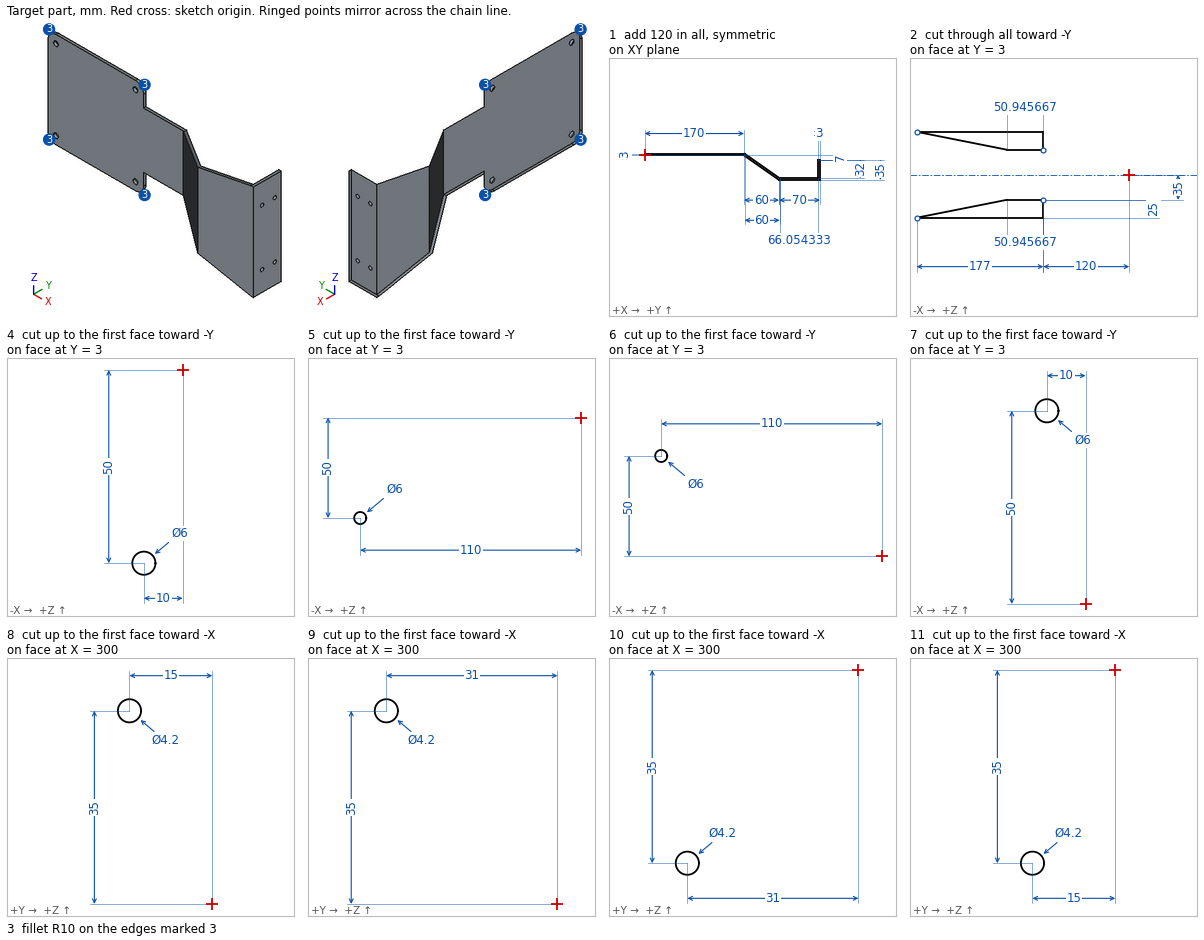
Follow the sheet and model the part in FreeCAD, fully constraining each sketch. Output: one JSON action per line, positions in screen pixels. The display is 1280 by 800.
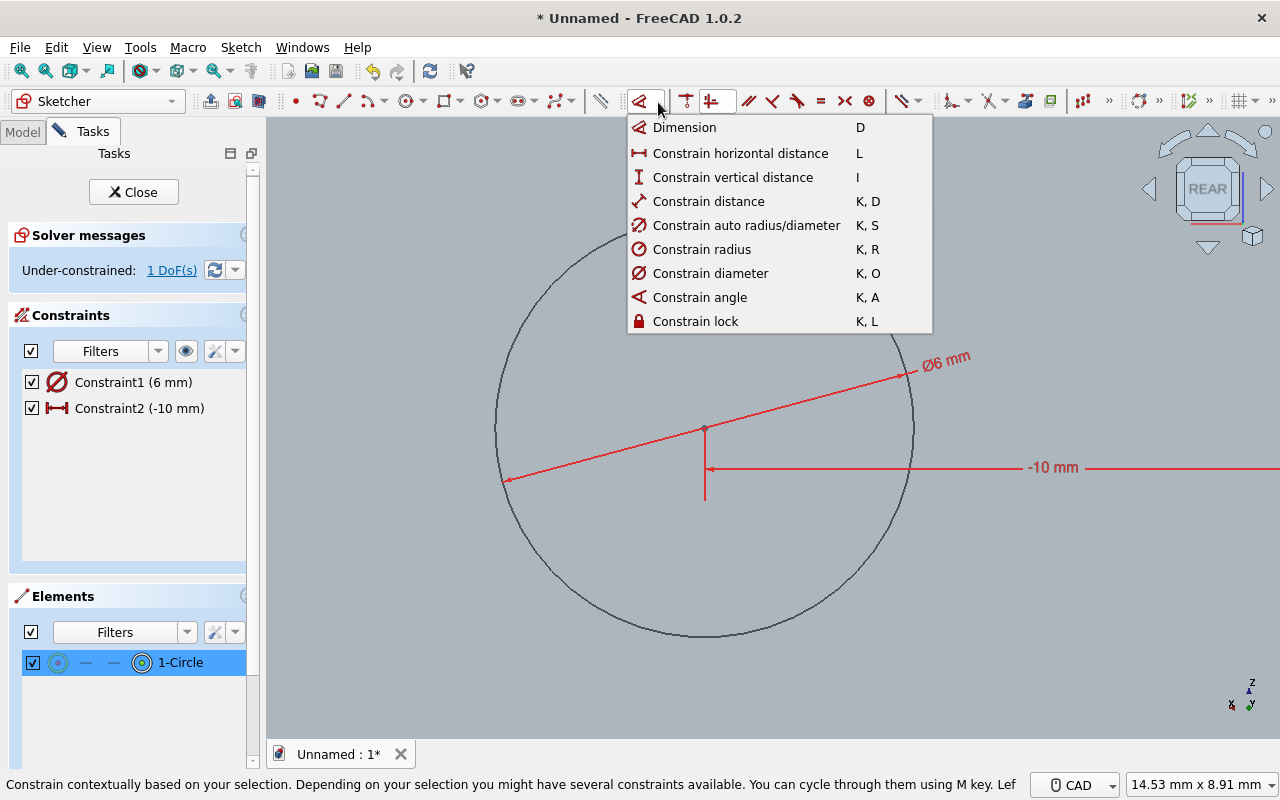
{"action": "left_click", "coordinate": [780, 177]}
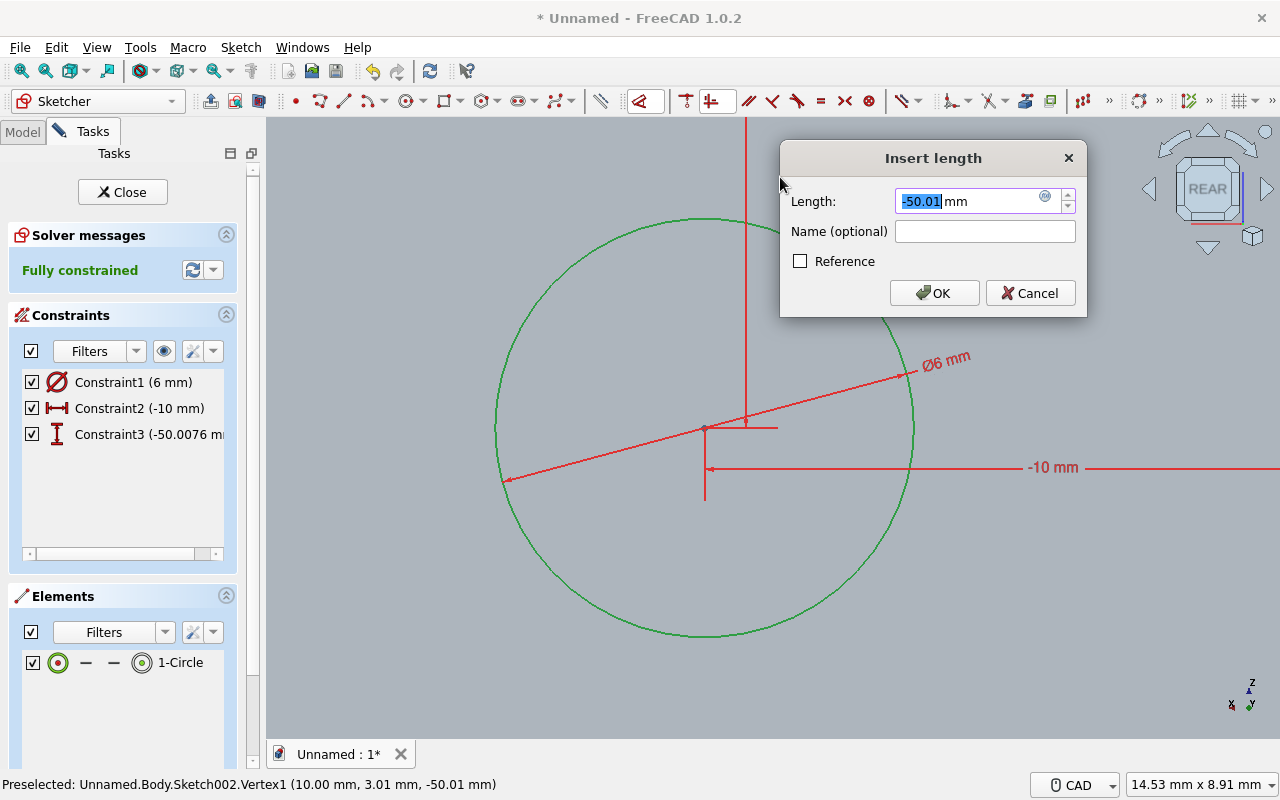
{"action": "type", "text": "-50"}
{"action": "key", "text": "Return"}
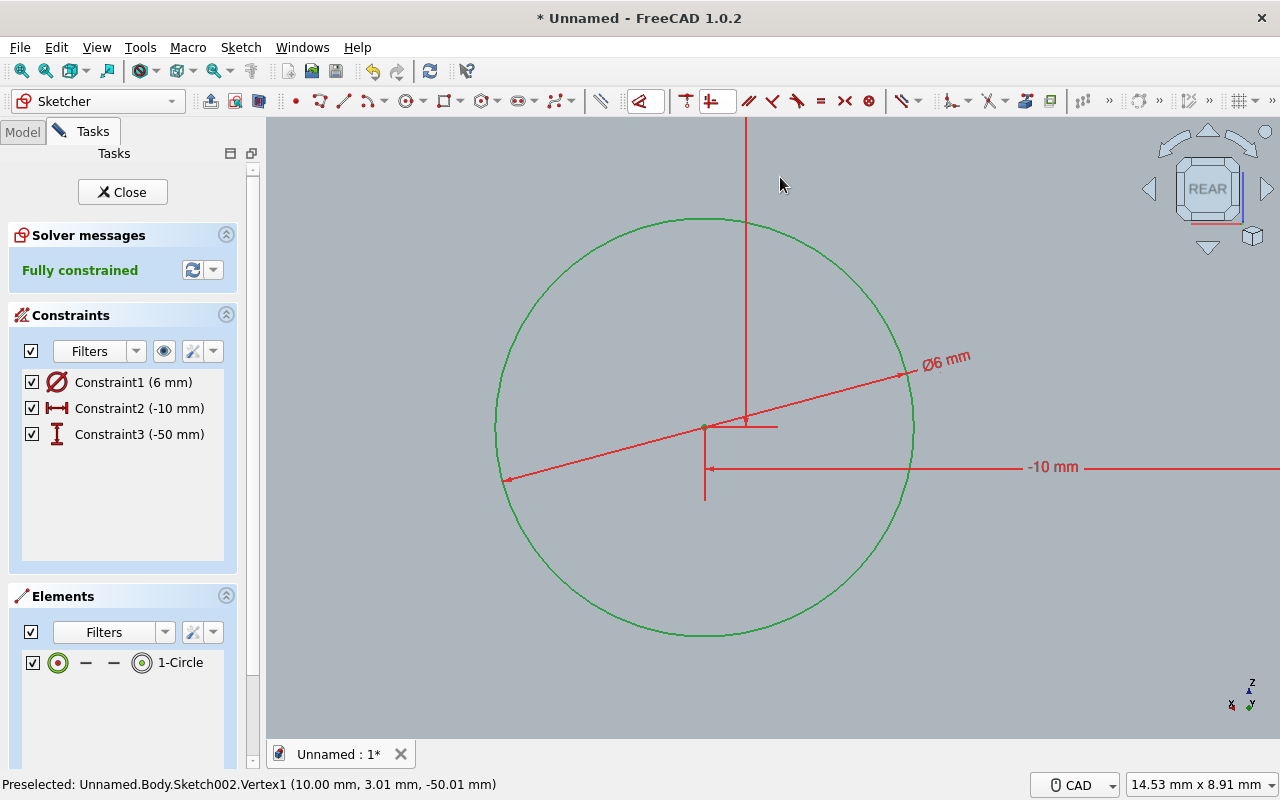
{"action": "left_click", "coordinate": [123, 192]}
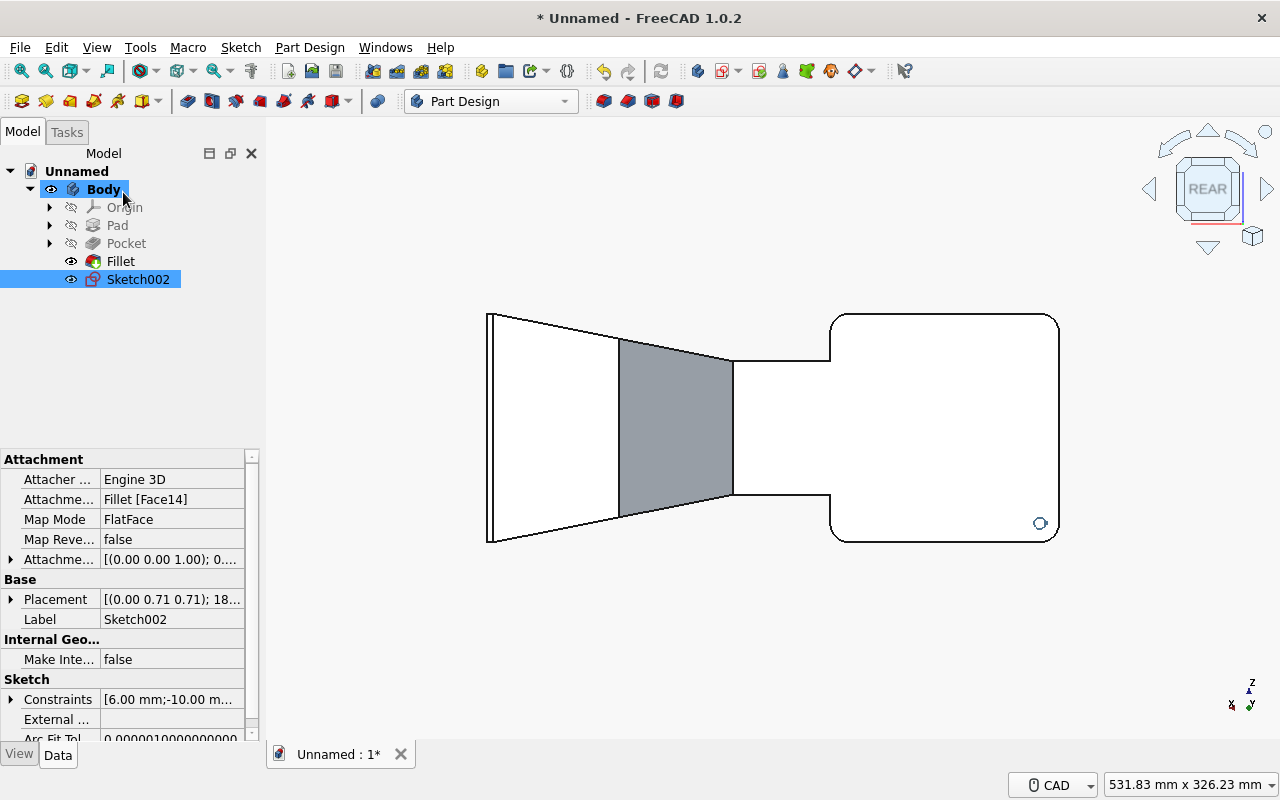
{"action": "left_click", "coordinate": [188, 102]}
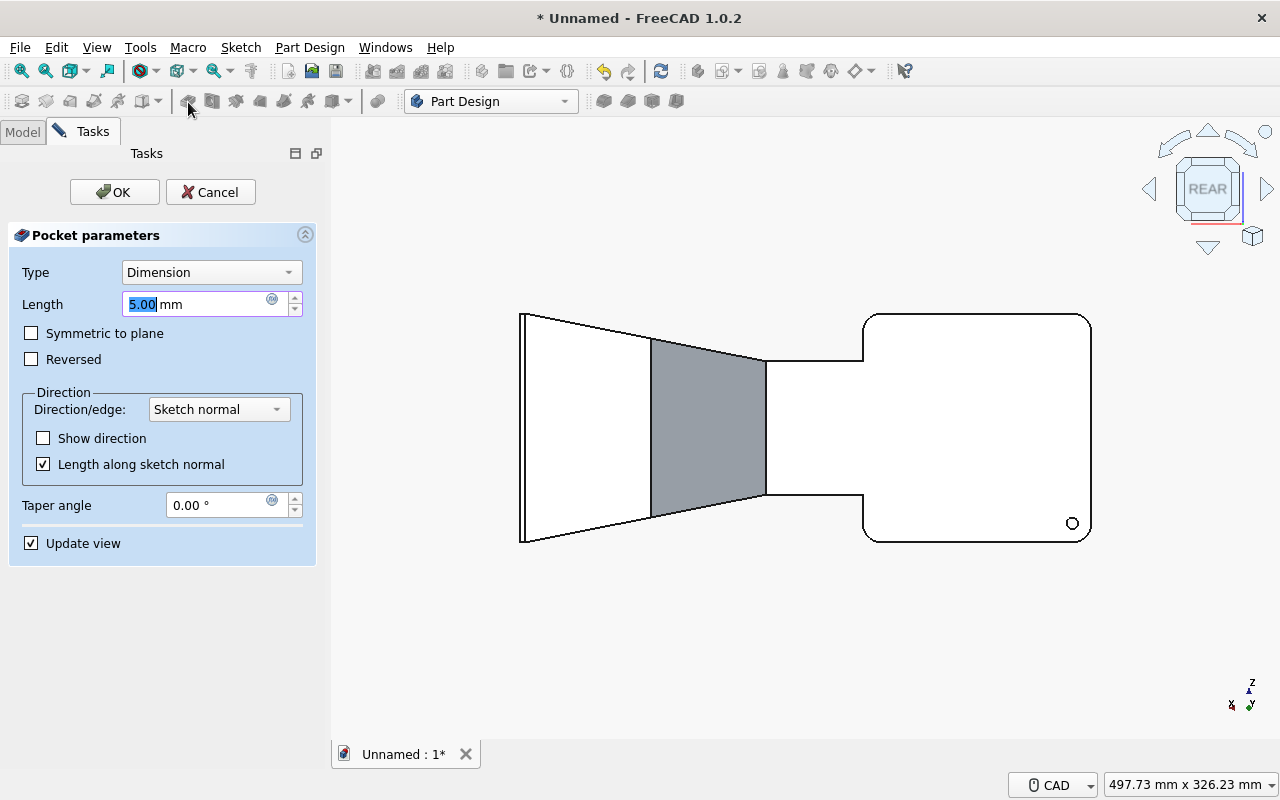
{"action": "left_click", "coordinate": [212, 272]}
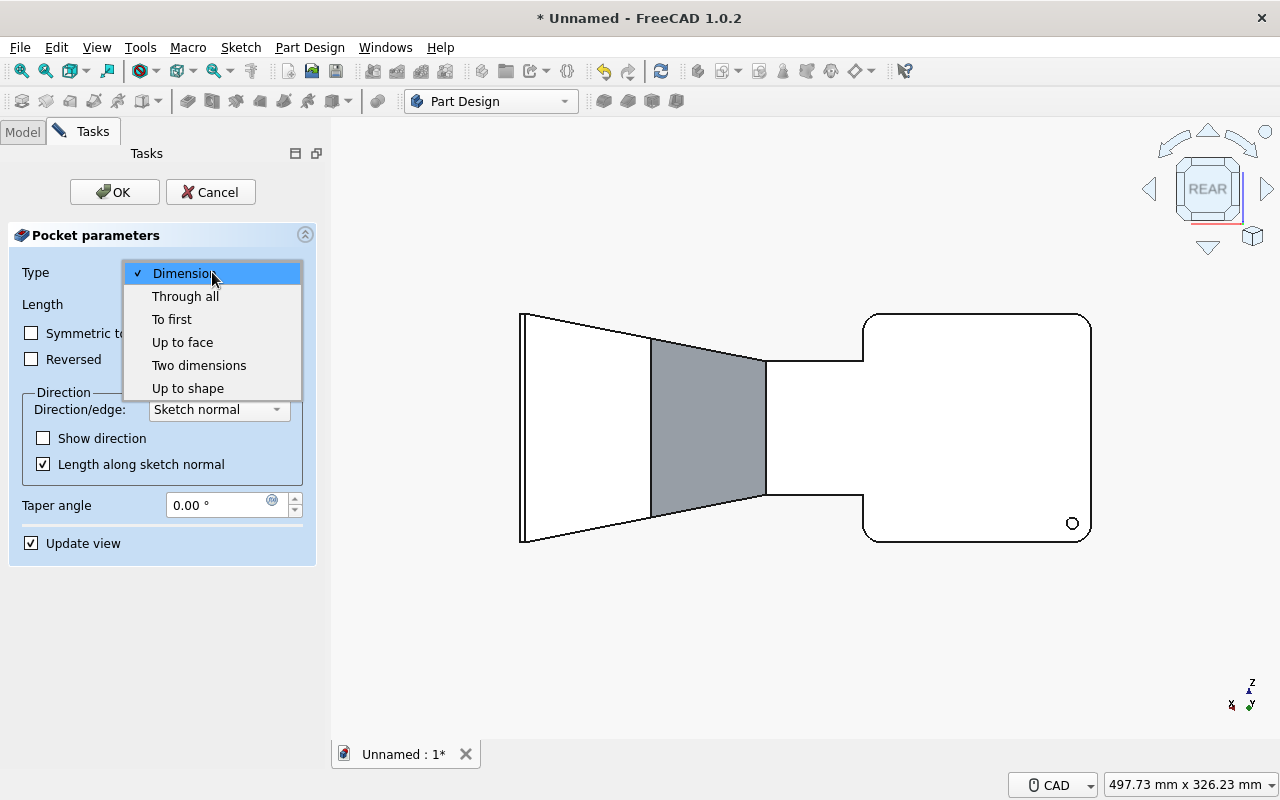
{"action": "left_click", "coordinate": [212, 320]}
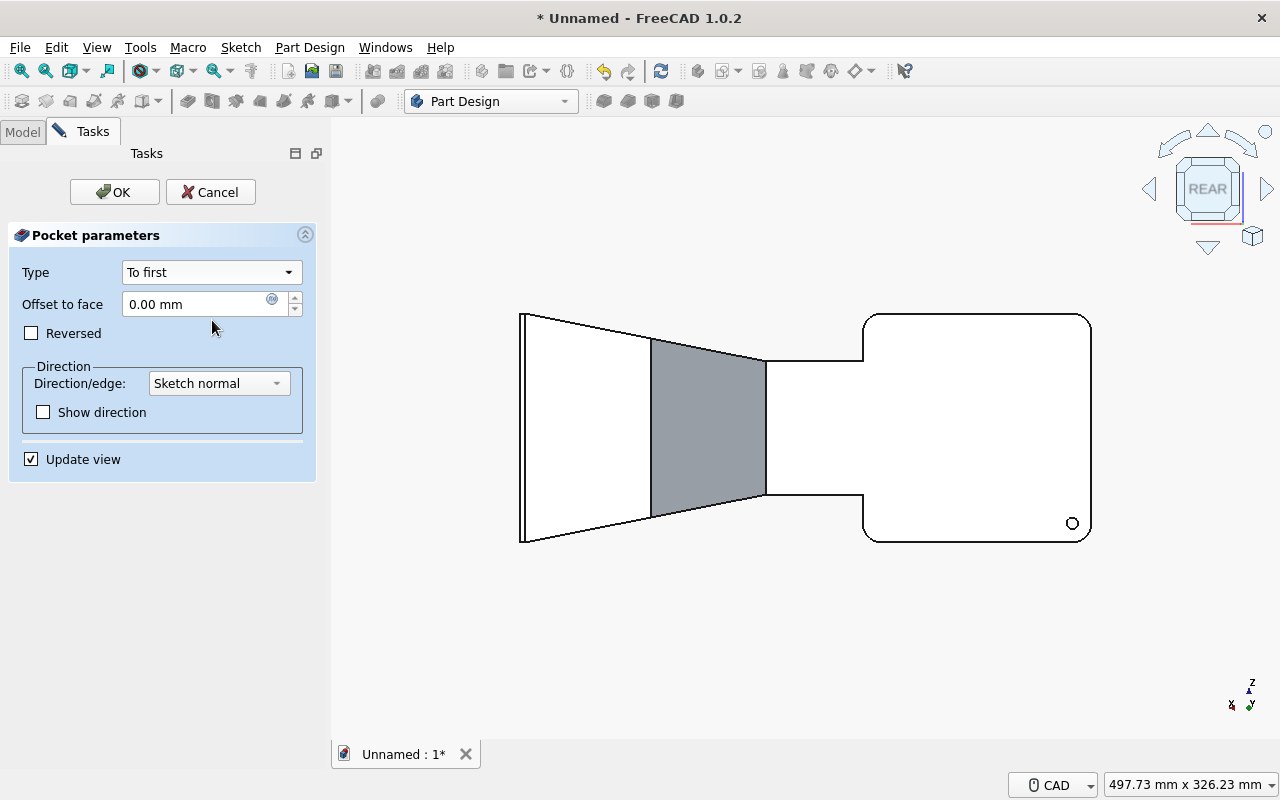
{"action": "left_click", "coordinate": [115, 192]}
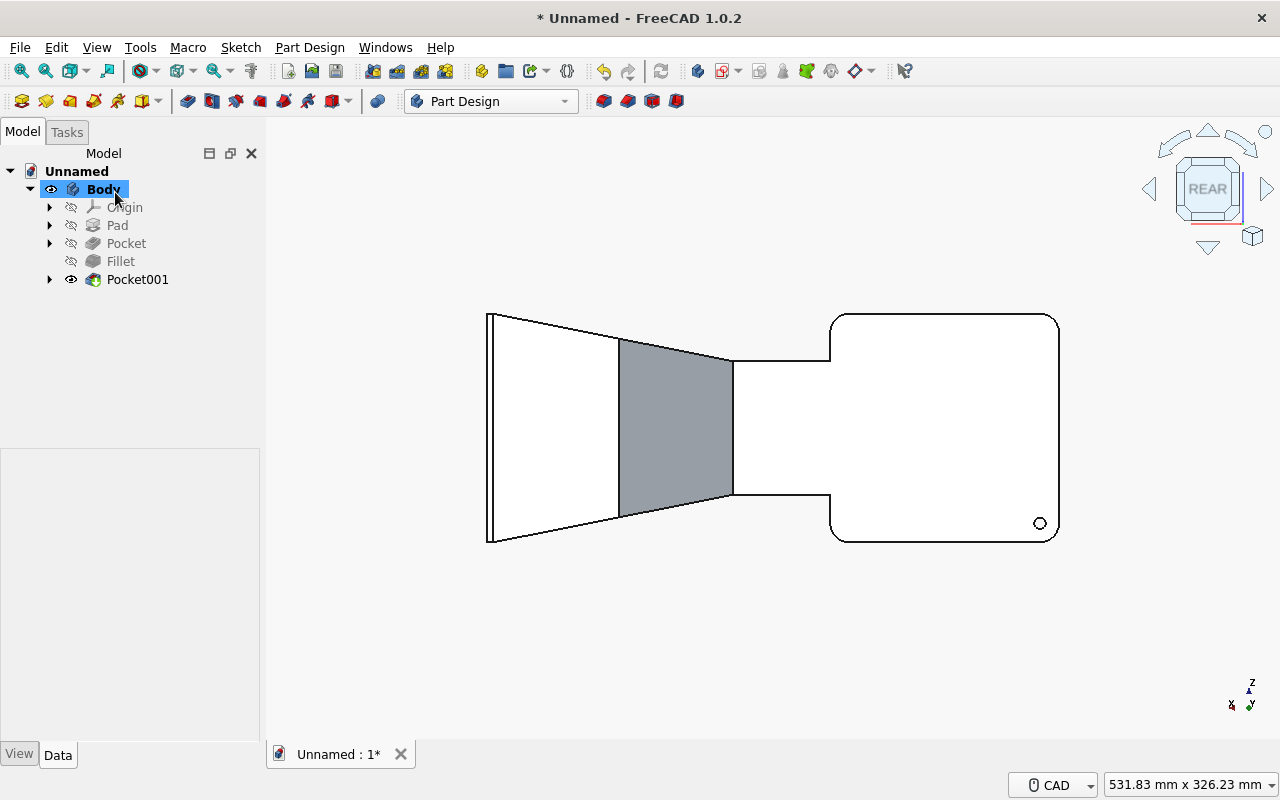
{"action": "left_click", "coordinate": [943, 427]}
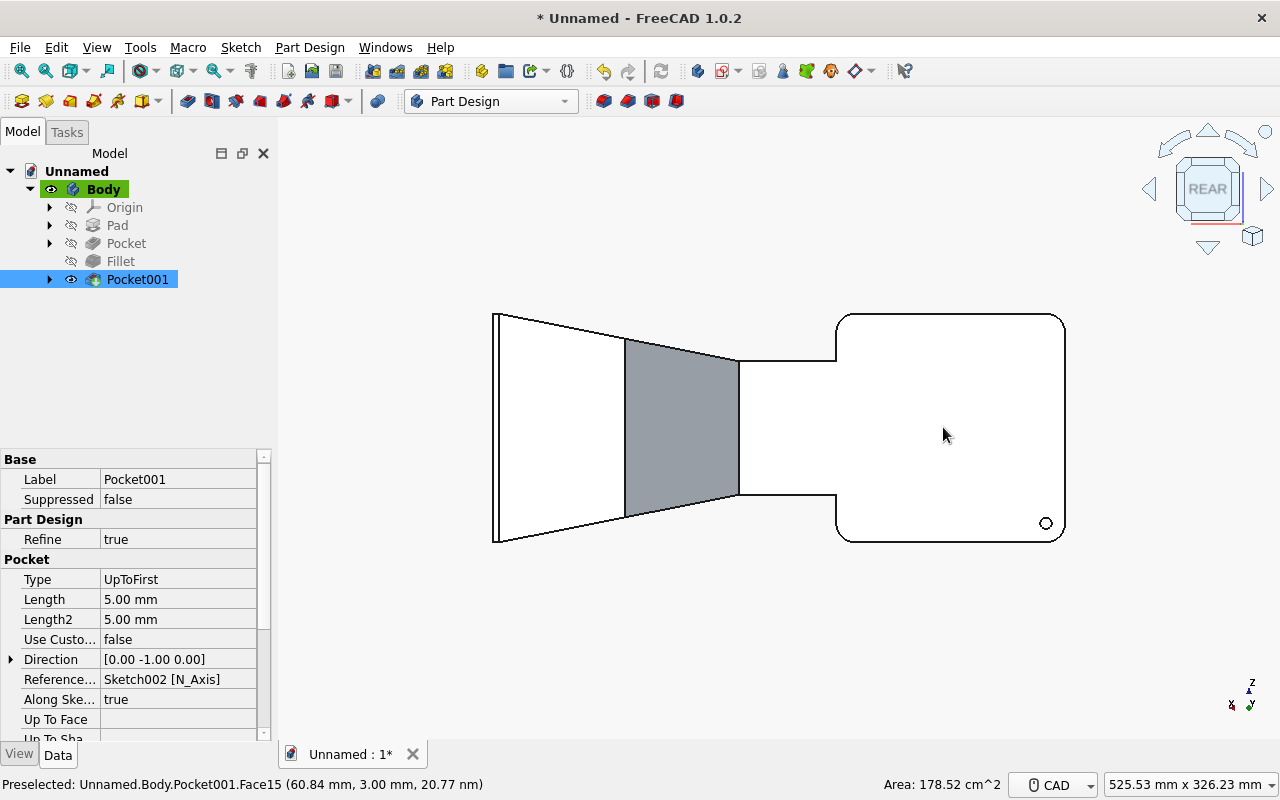
{"action": "left_click", "coordinate": [722, 72]}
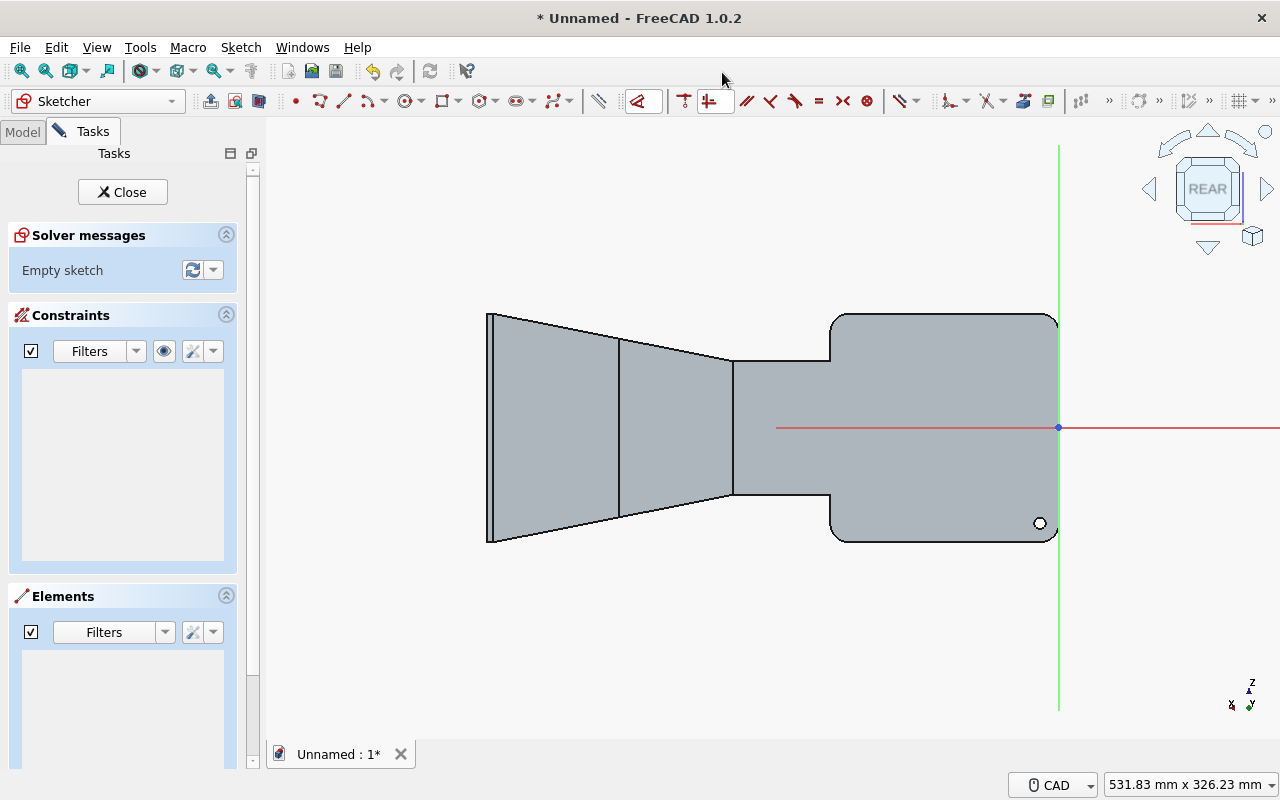
{"action": "scroll", "coordinate": [857, 528], "scroll_direction": "up", "scroll_amount": 15}